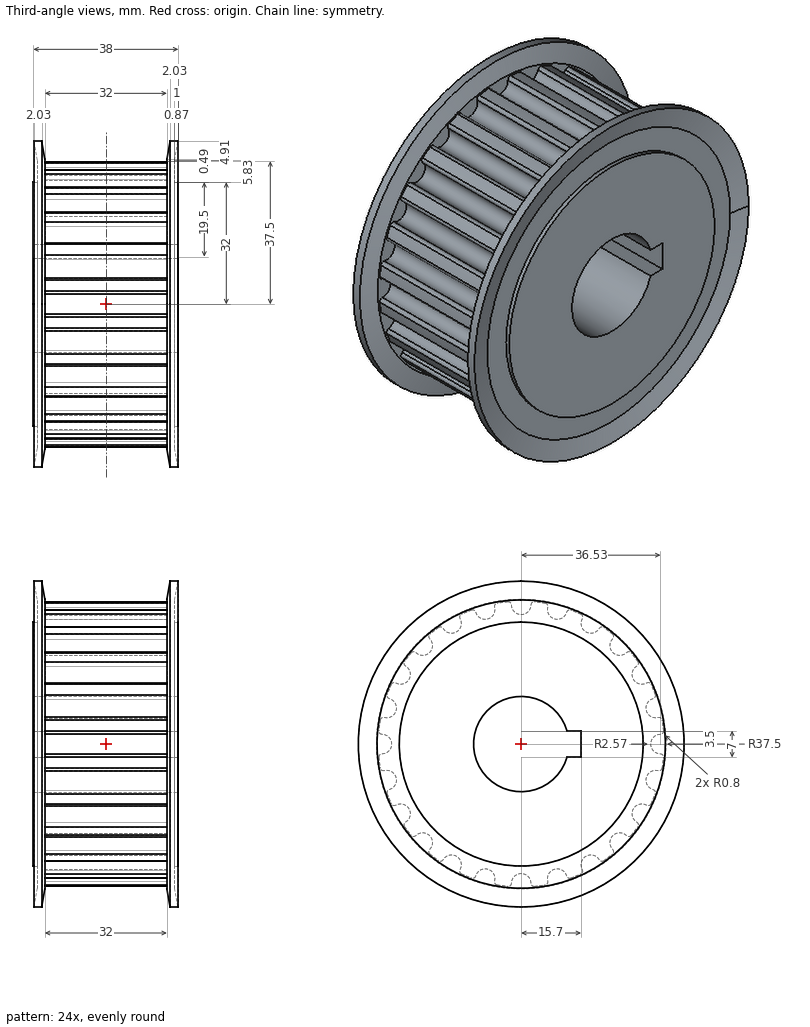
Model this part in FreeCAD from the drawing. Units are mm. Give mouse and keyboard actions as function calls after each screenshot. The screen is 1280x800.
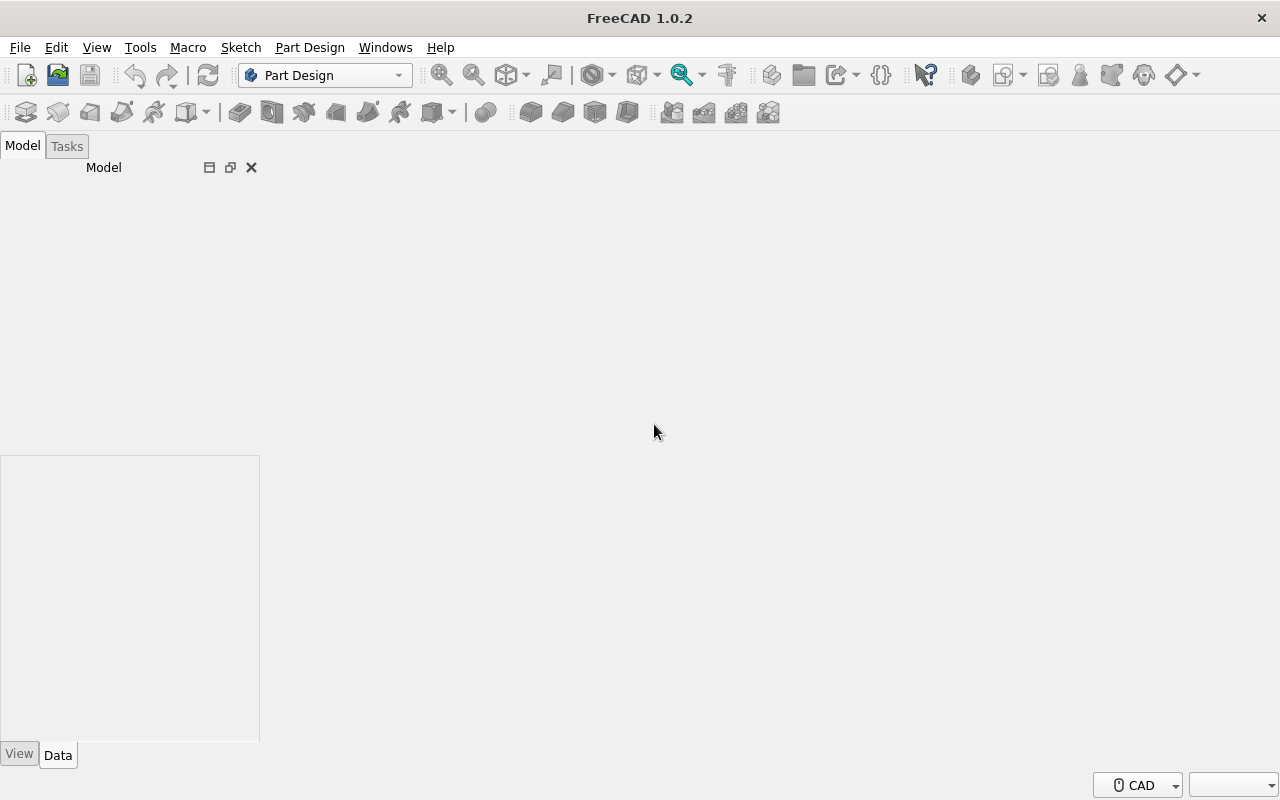
click(26, 76)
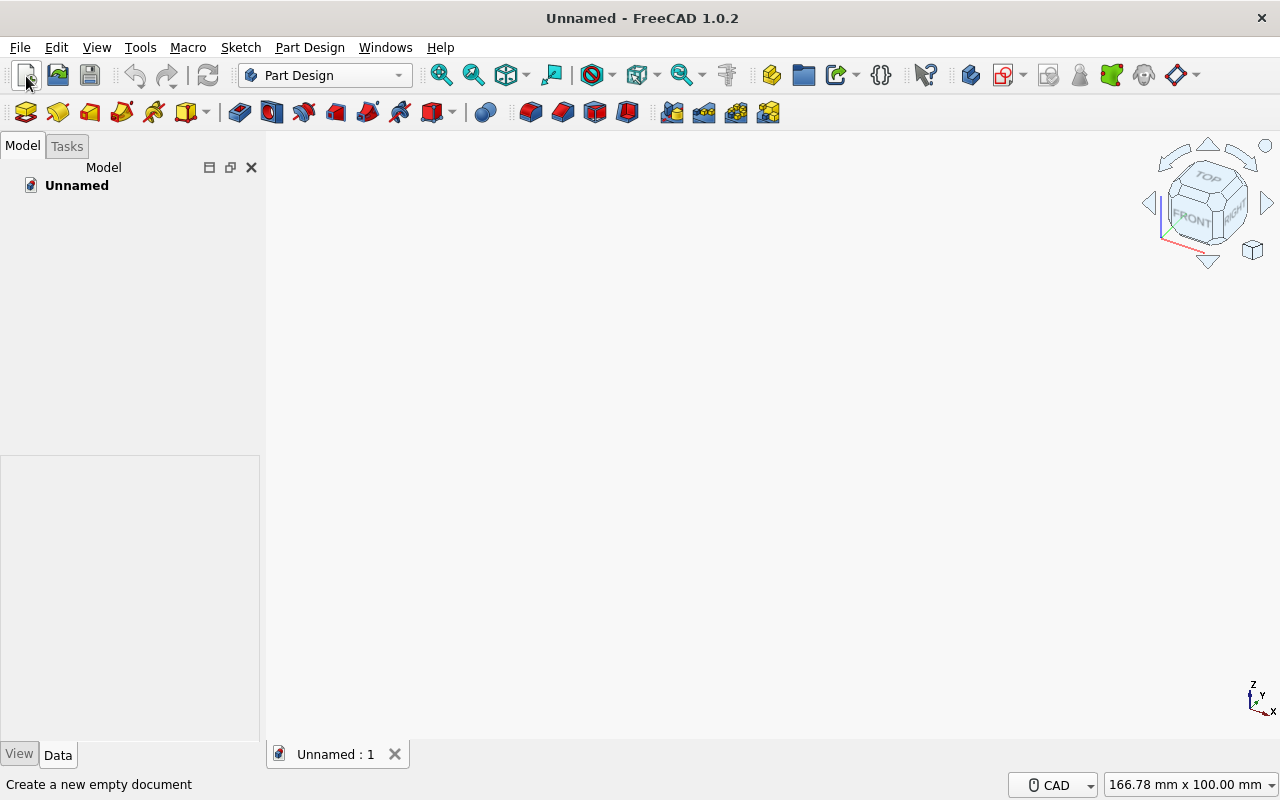
click(1004, 76)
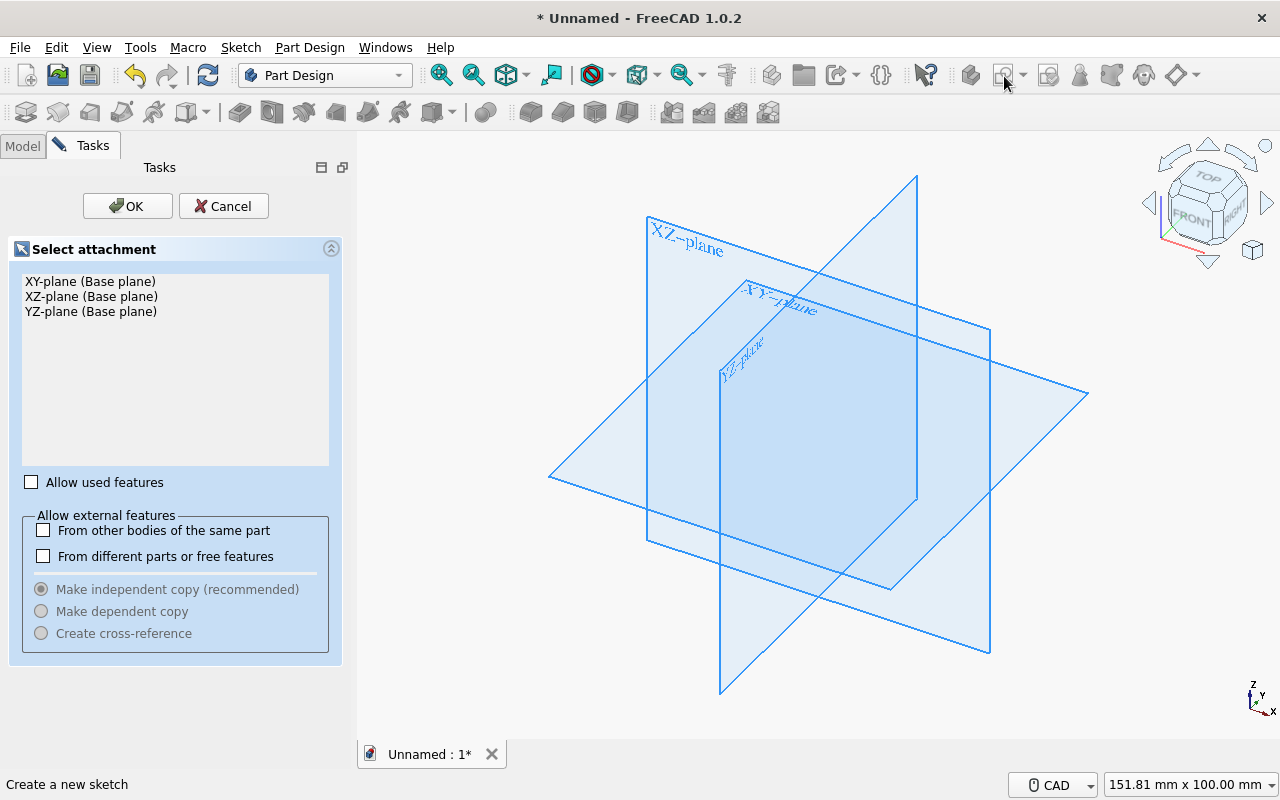
click(82, 282)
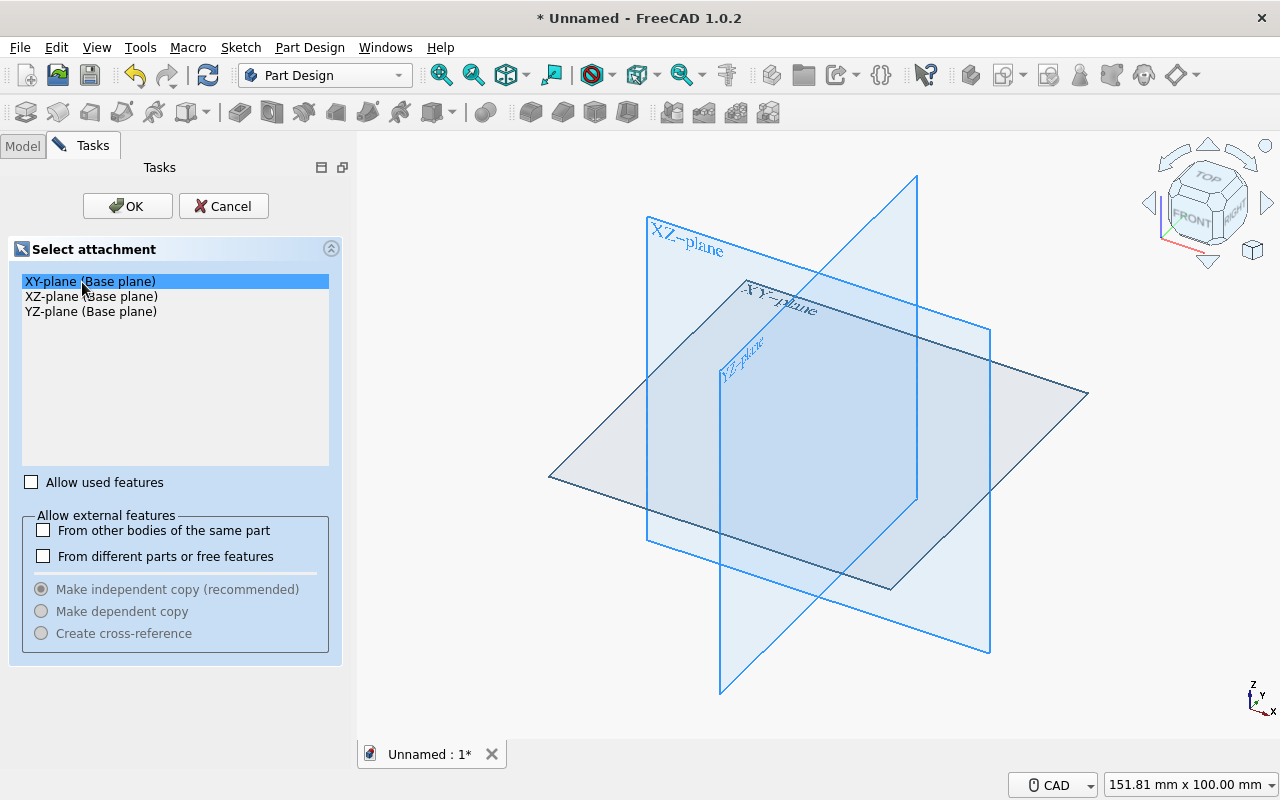
click(128, 206)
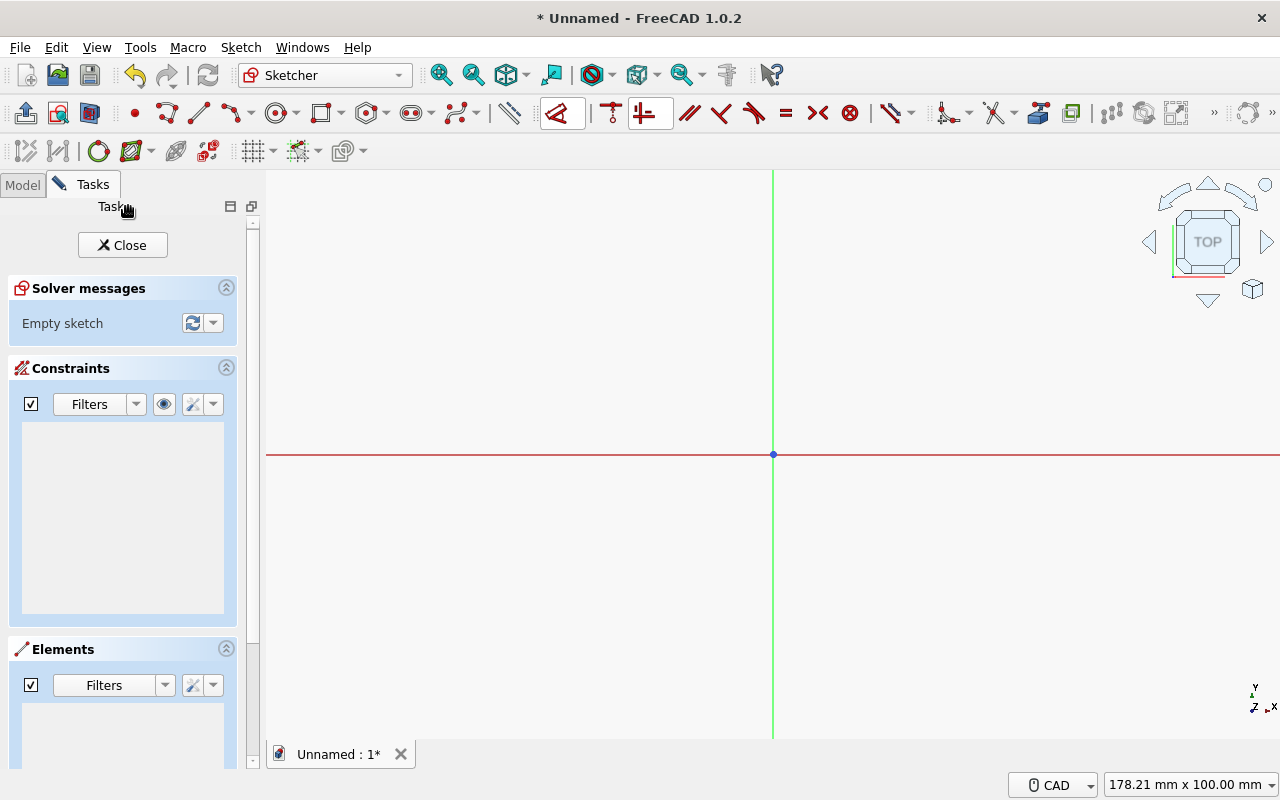
scroll(395, 711, down, 1)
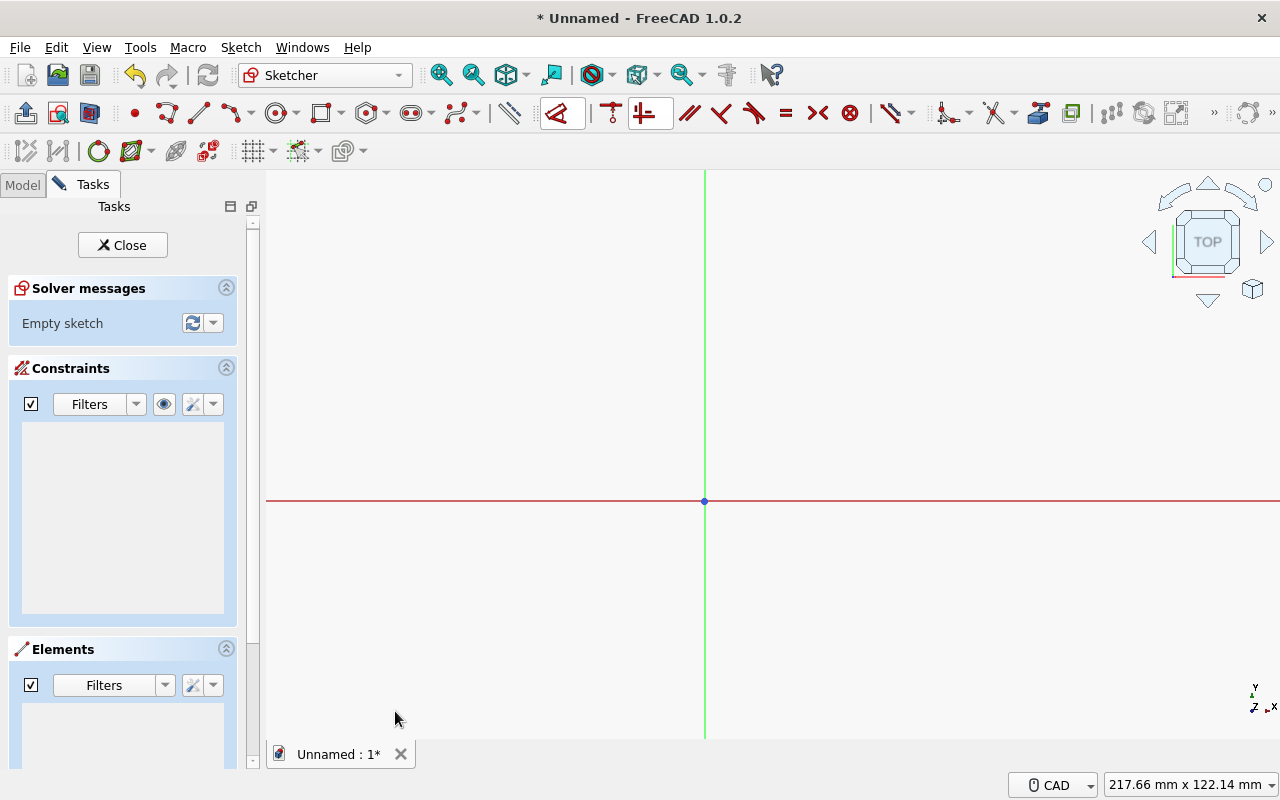
scroll(705, 337, up, 3)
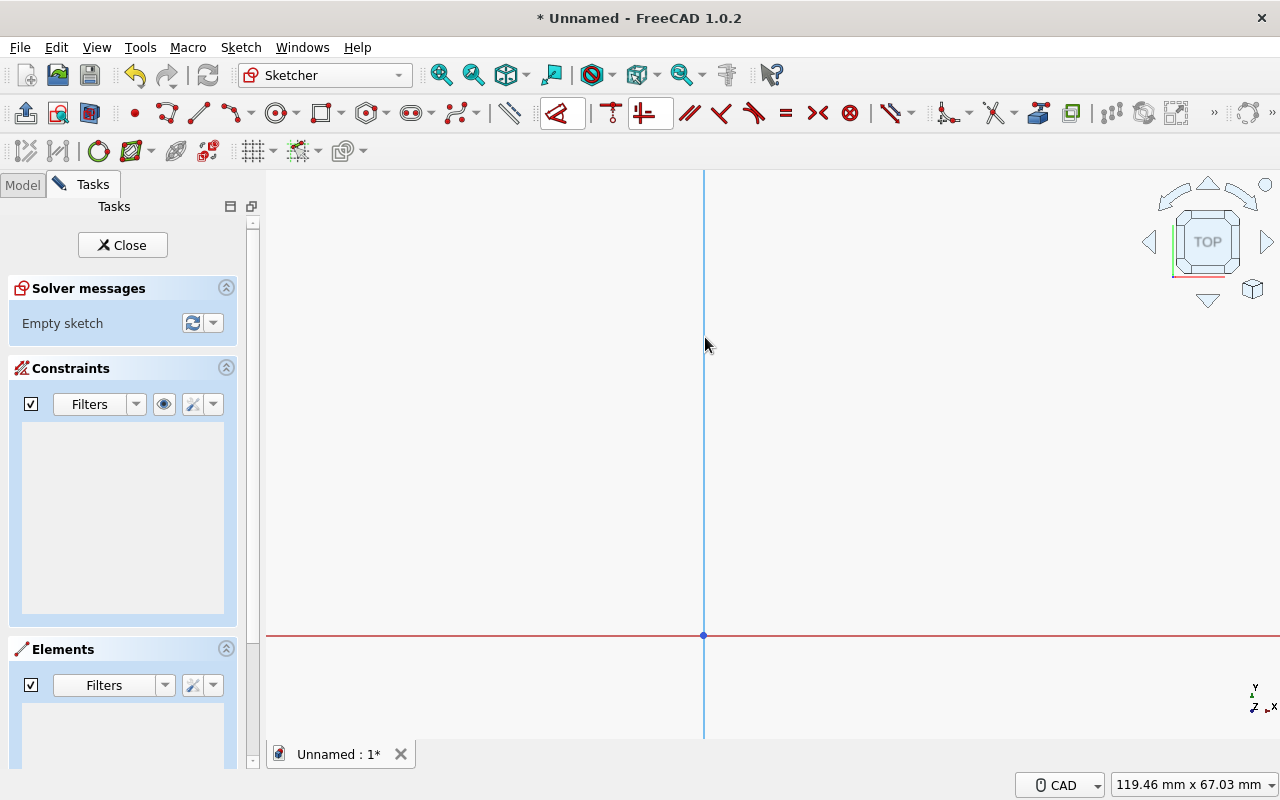
click(168, 114)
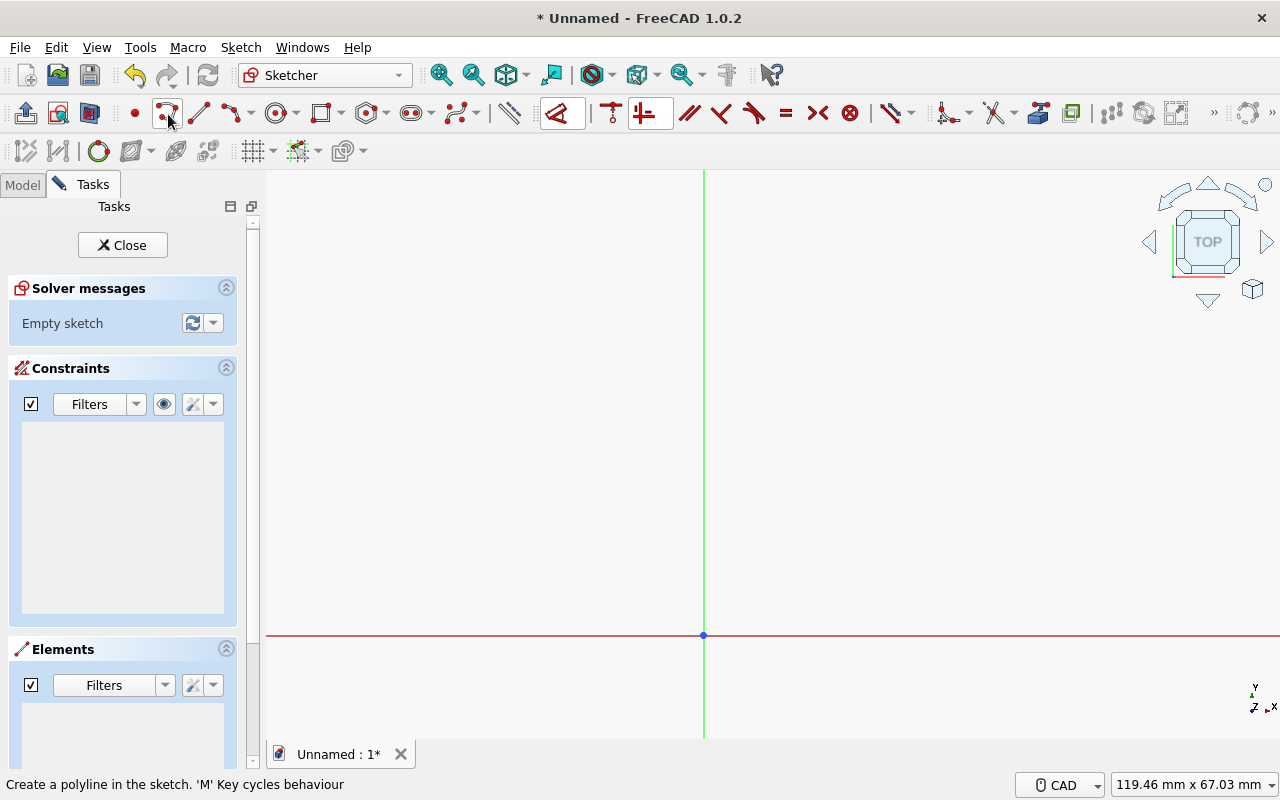
click(542, 530)
click(865, 530)
click(865, 364)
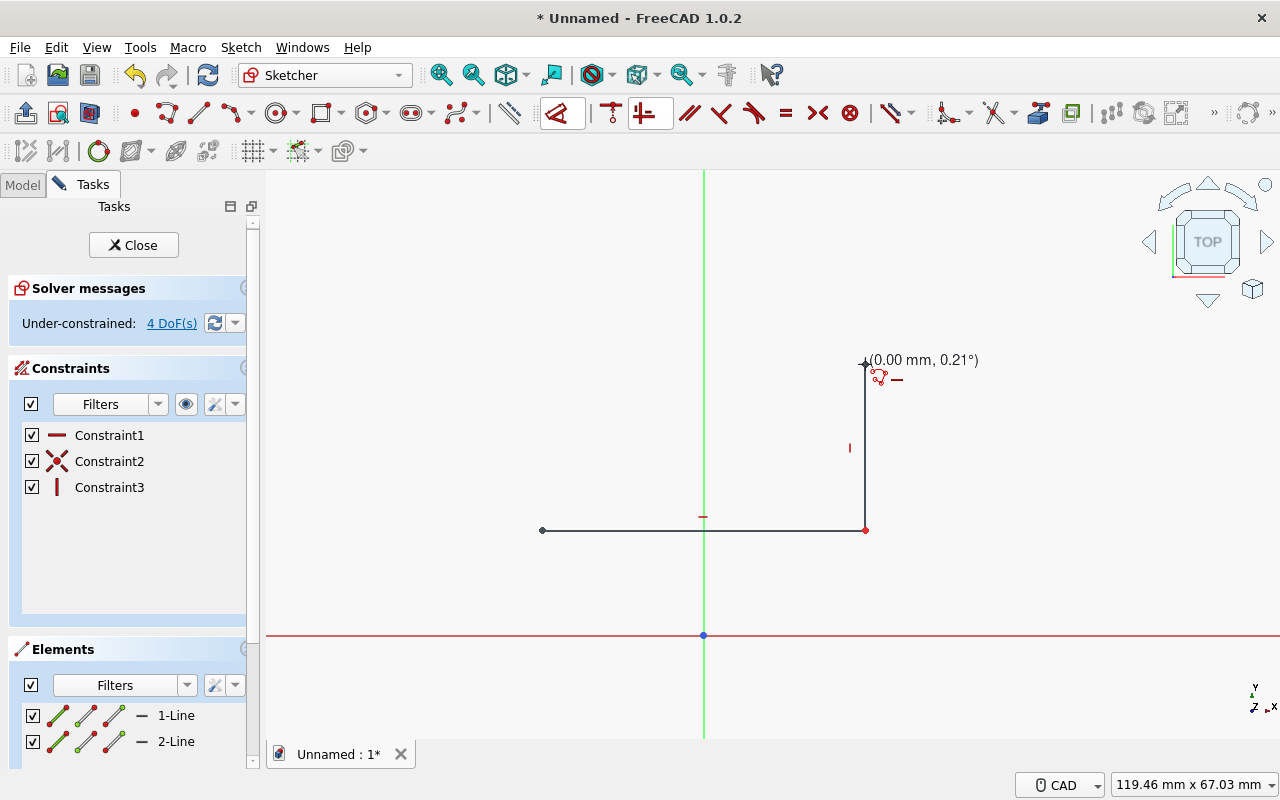
scroll(857, 364, up, 4)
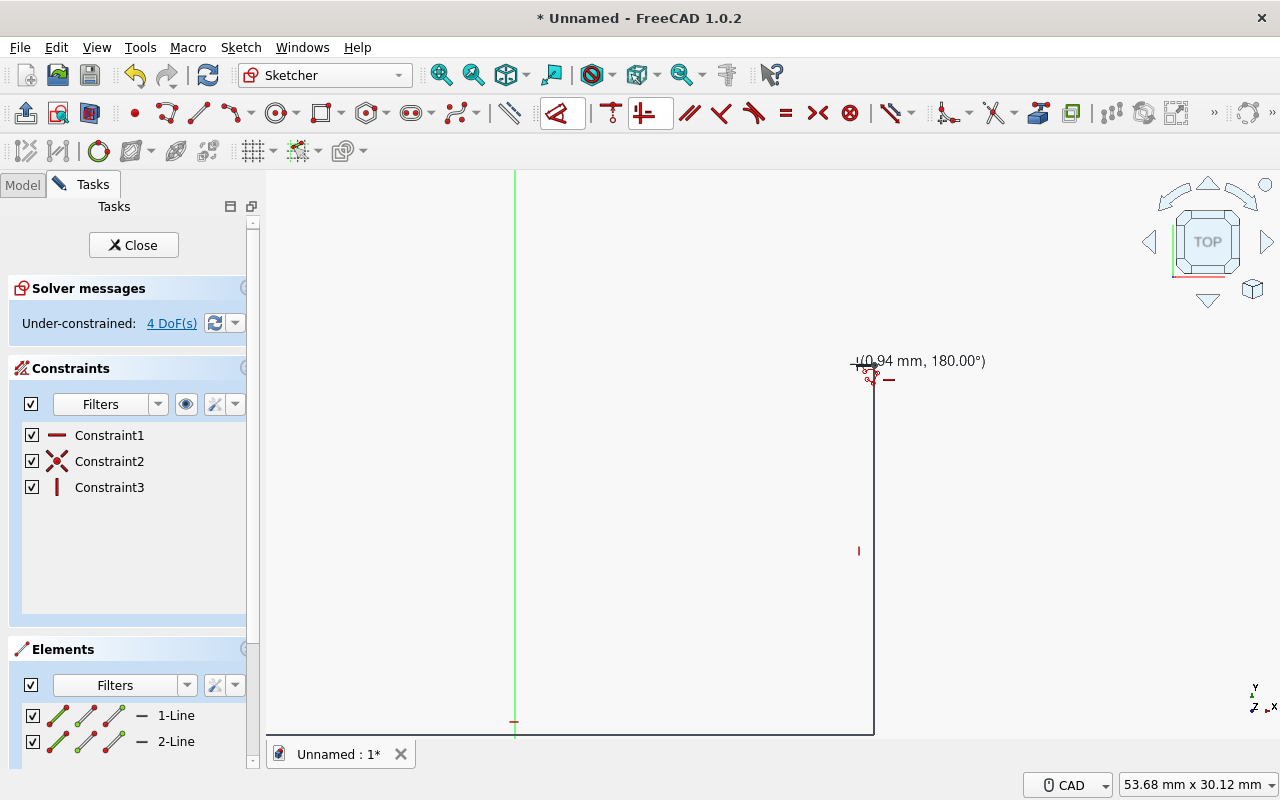
click(855, 364)
click(855, 254)